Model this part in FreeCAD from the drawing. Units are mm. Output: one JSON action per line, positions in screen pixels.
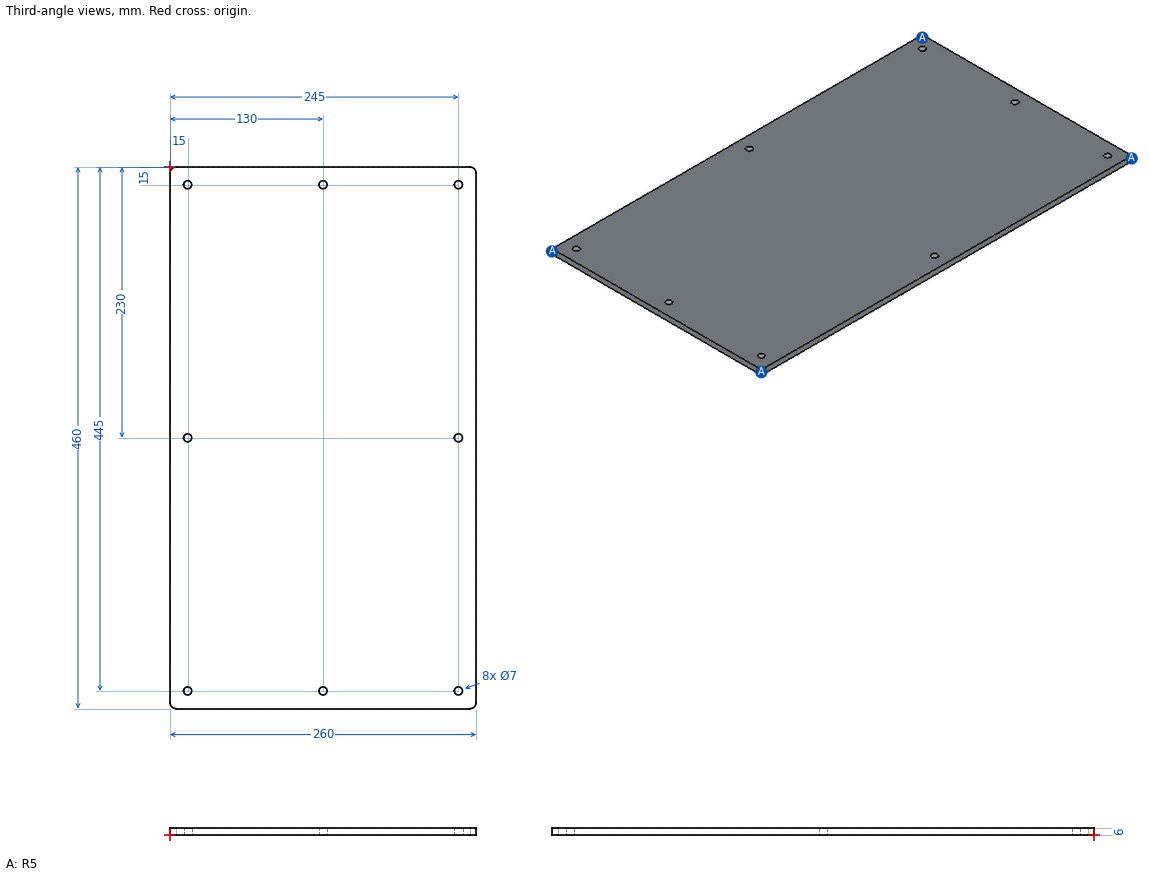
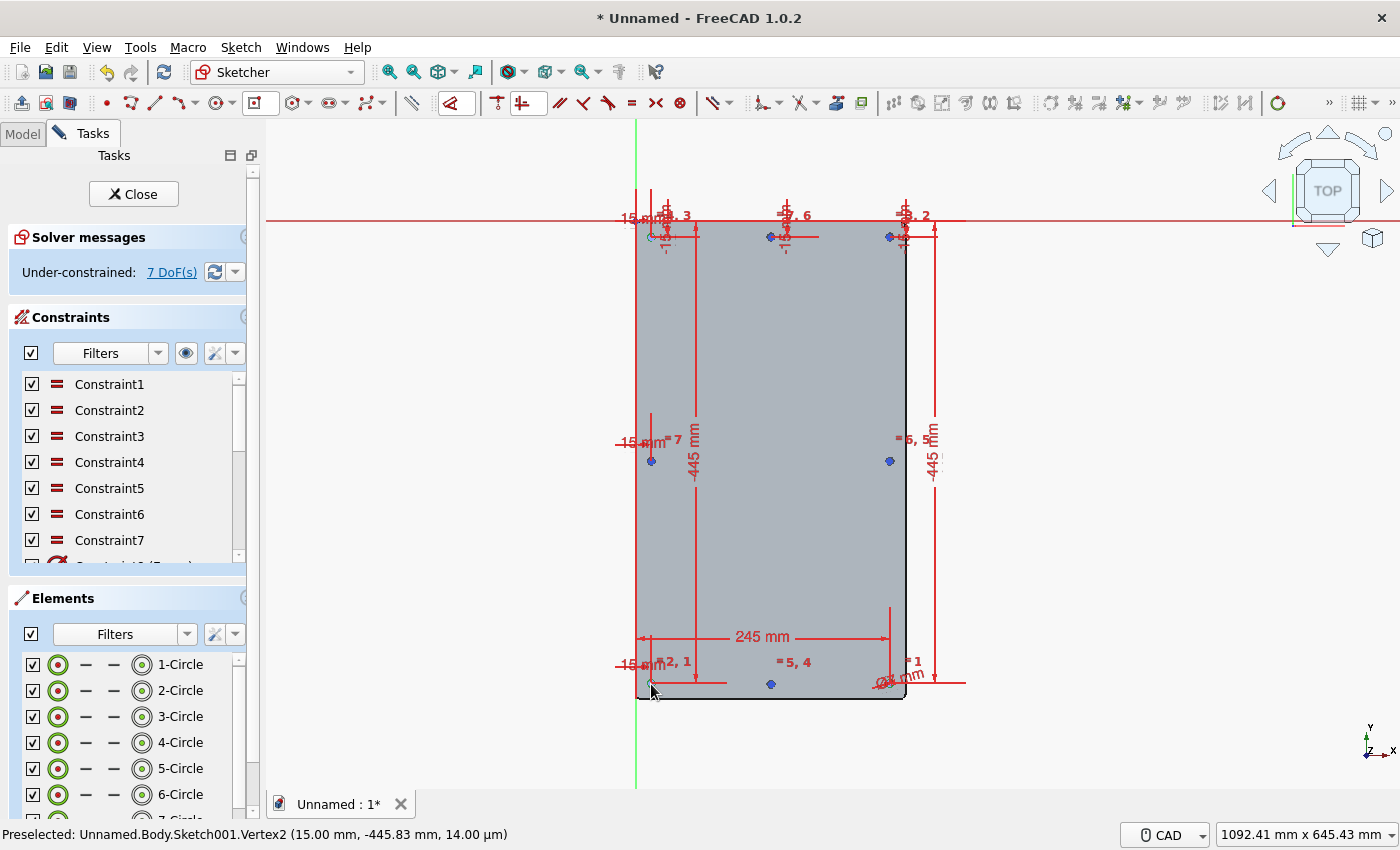
{"action": "left_click", "coordinate": [890, 237]}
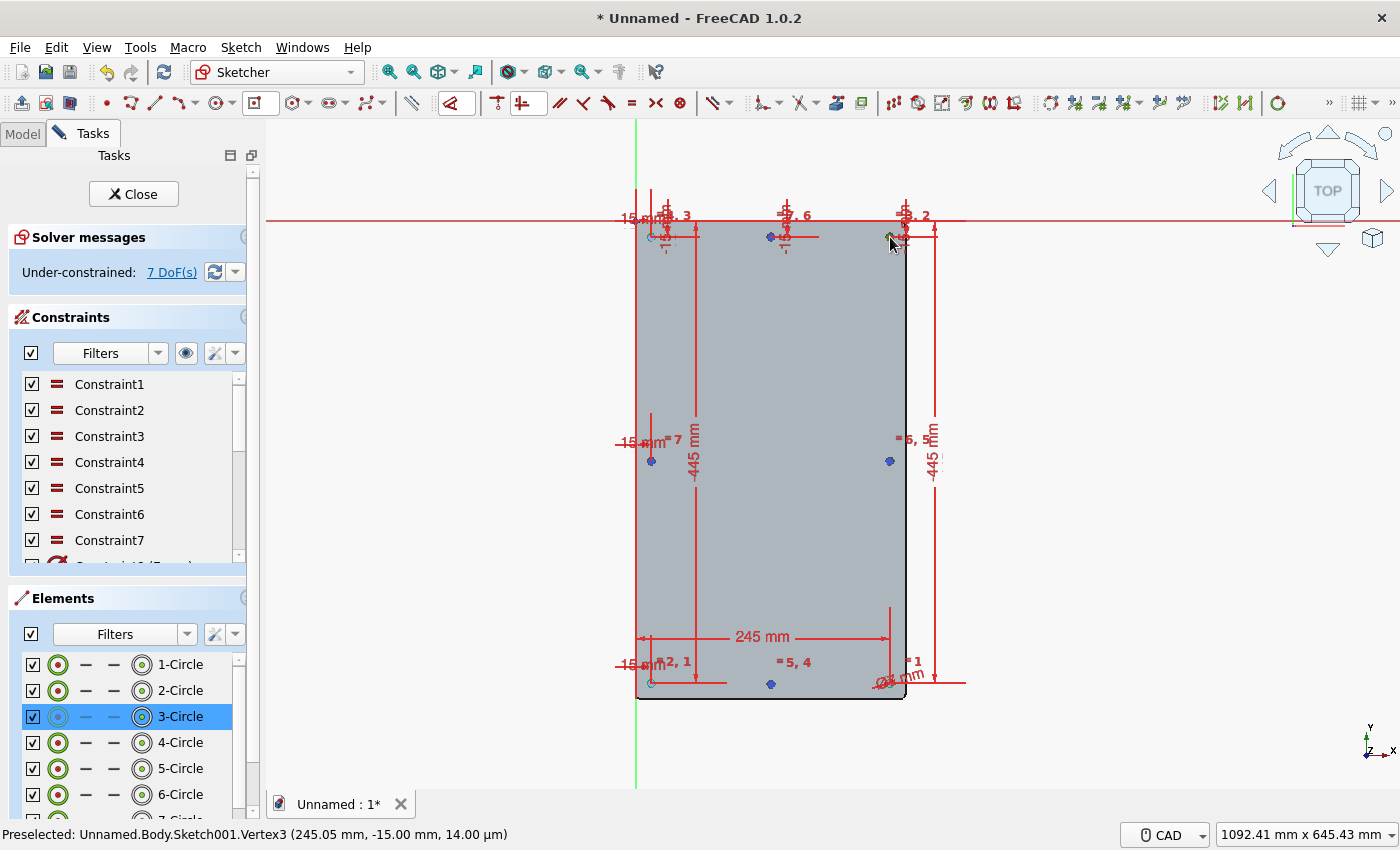
{"action": "key", "text": "l"}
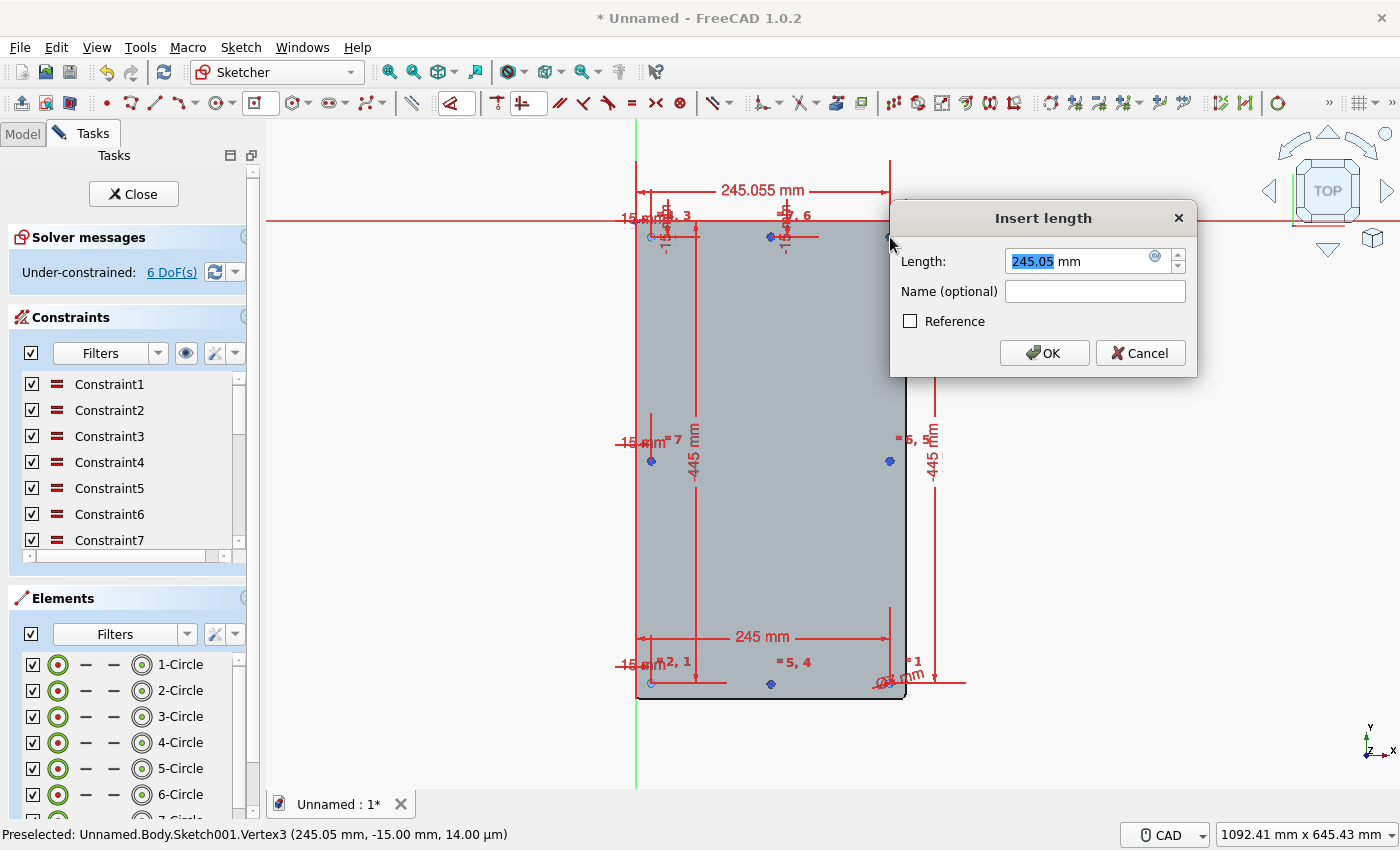
{"action": "type", "text": "245"}
{"action": "key", "text": "Return"}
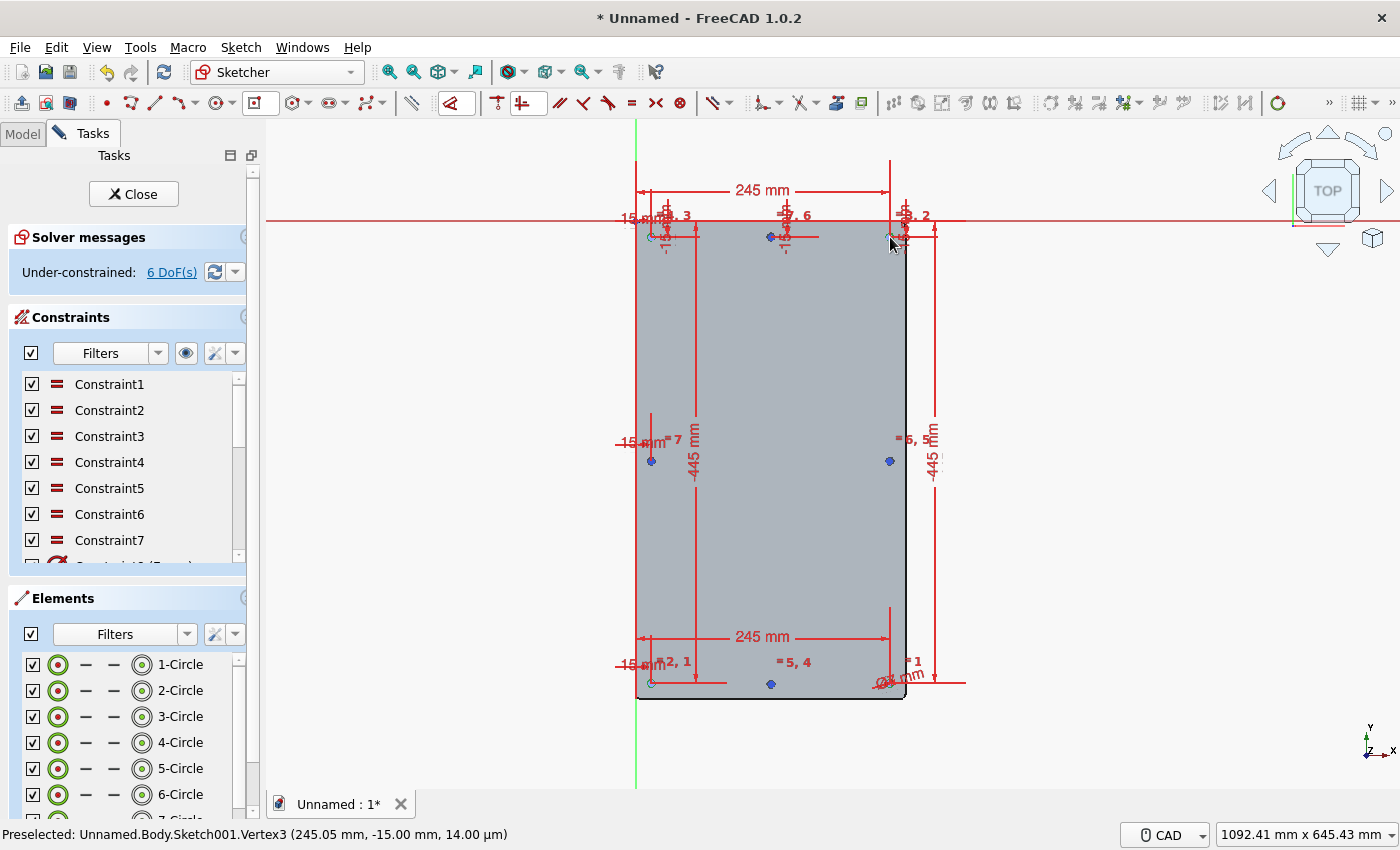
{"action": "left_click", "coordinate": [771, 684]}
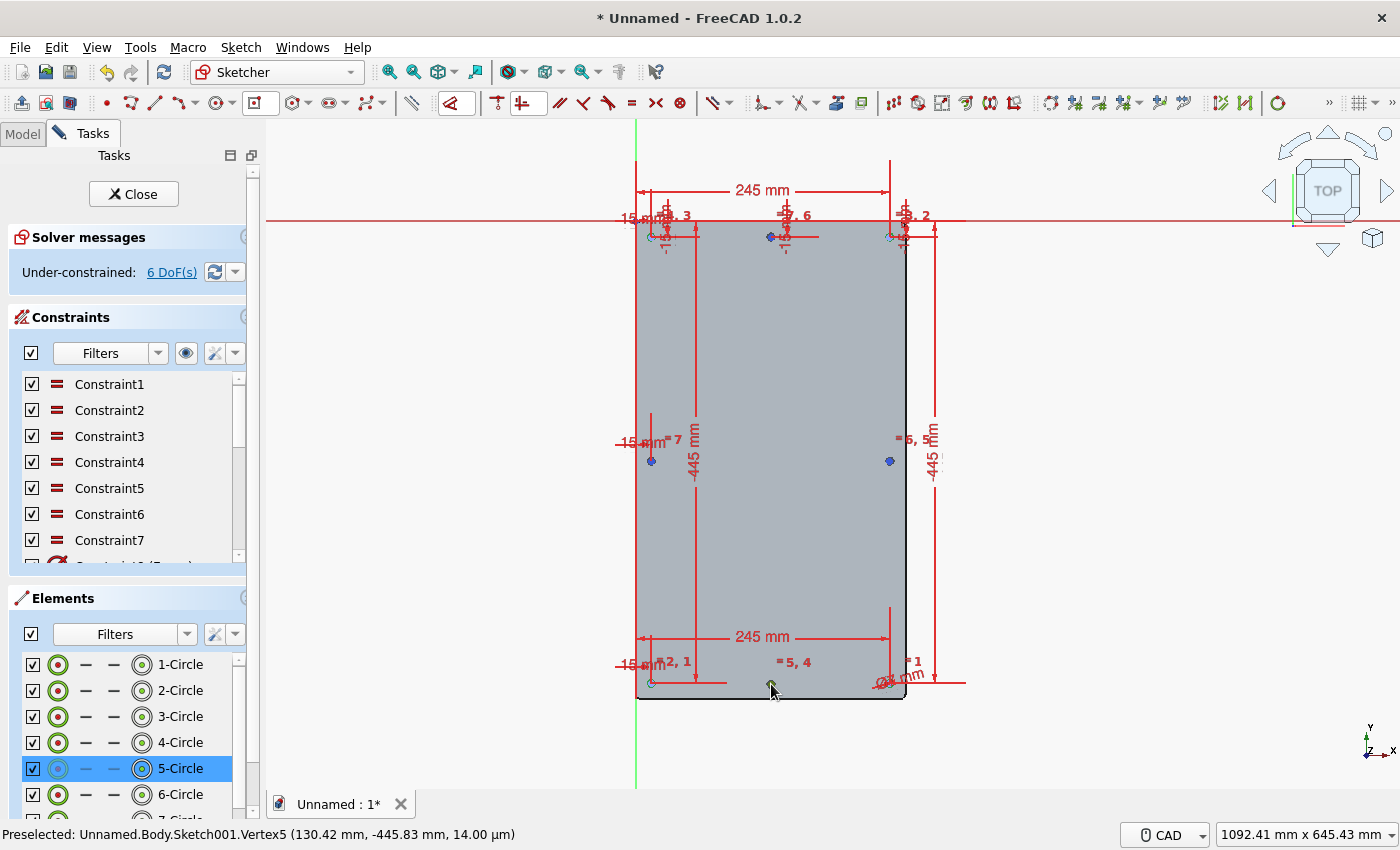
{"action": "key", "text": "l"}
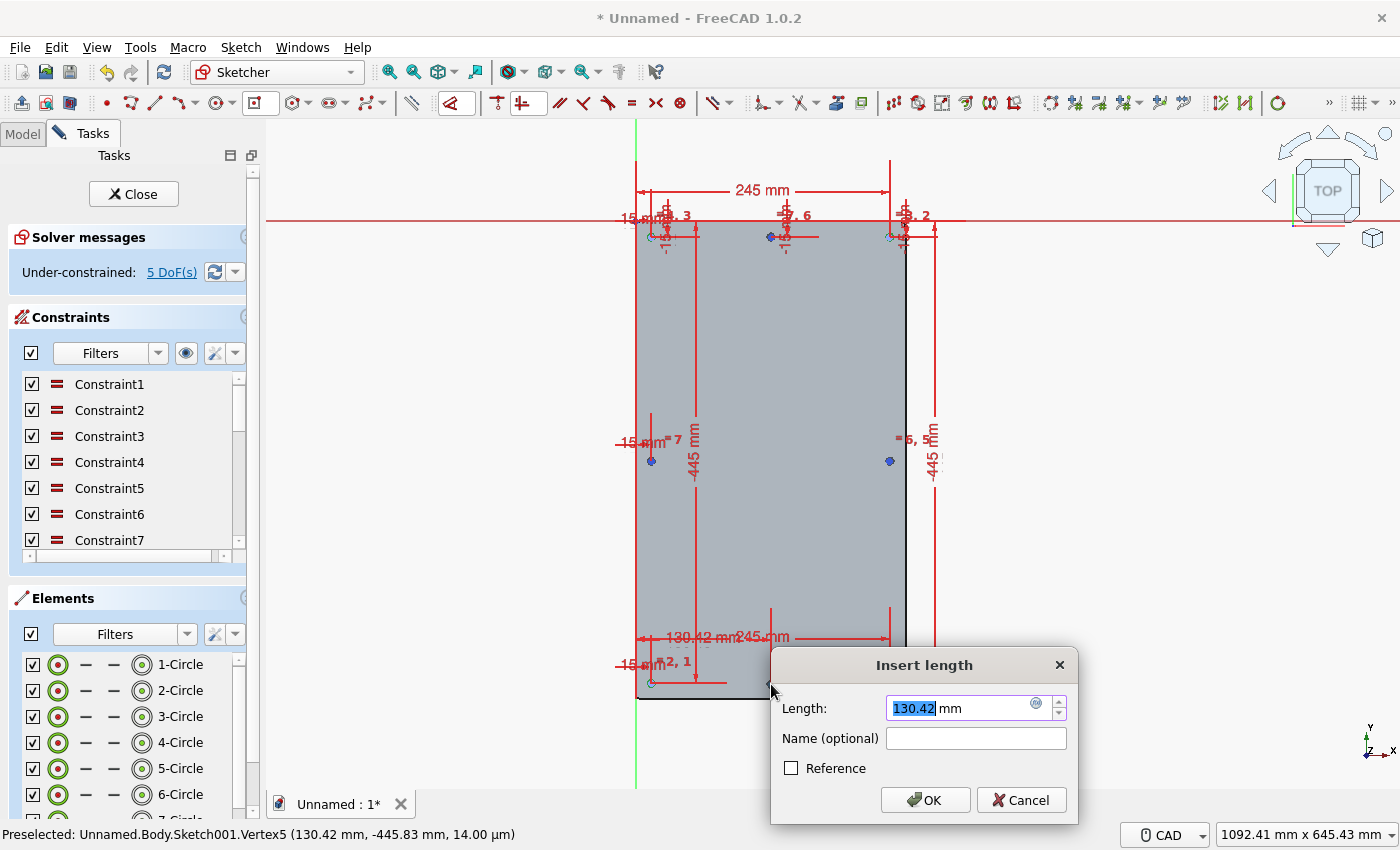
{"action": "type", "text": "130"}
{"action": "key", "text": "Return"}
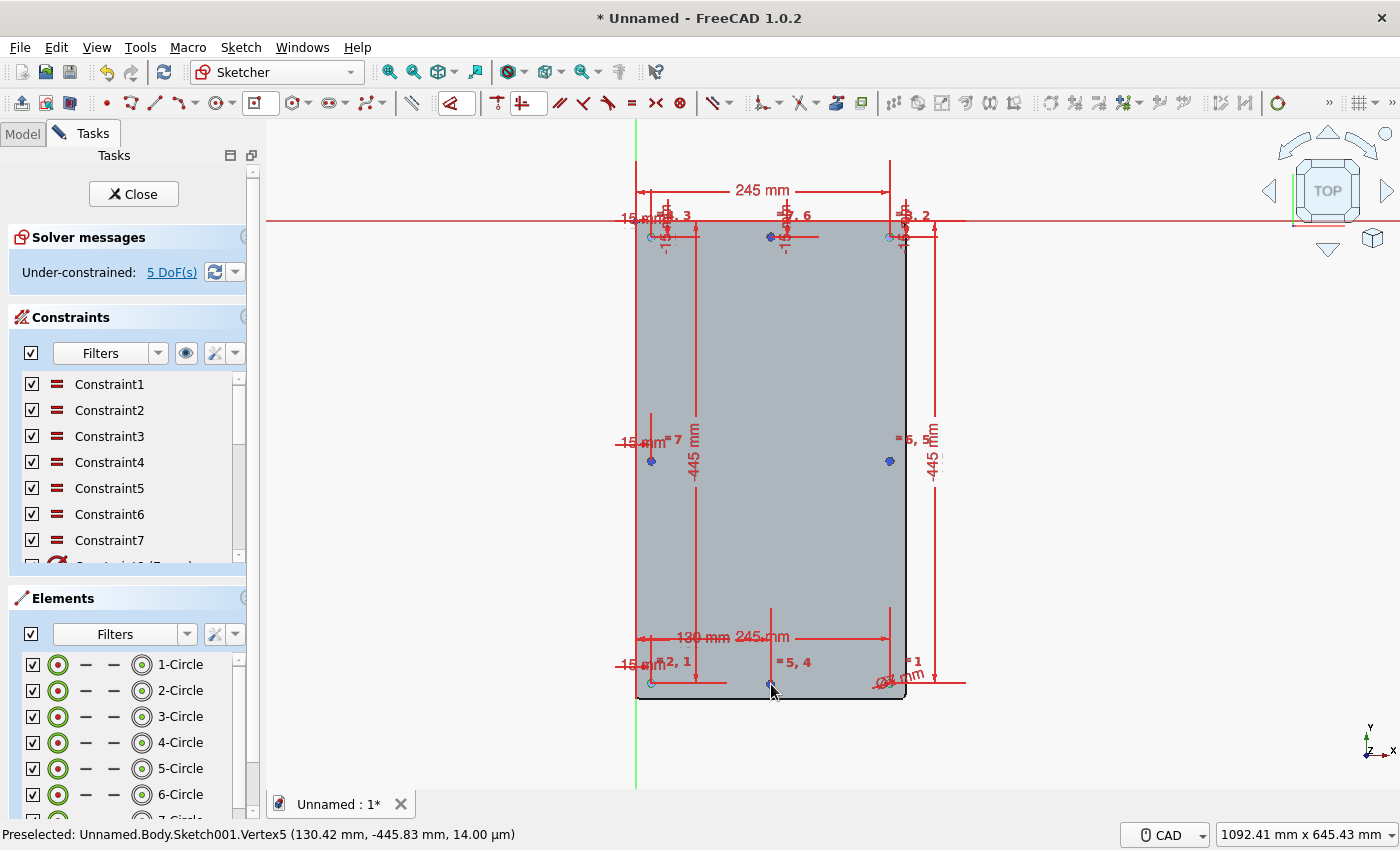
{"action": "left_click", "coordinate": [771, 684]}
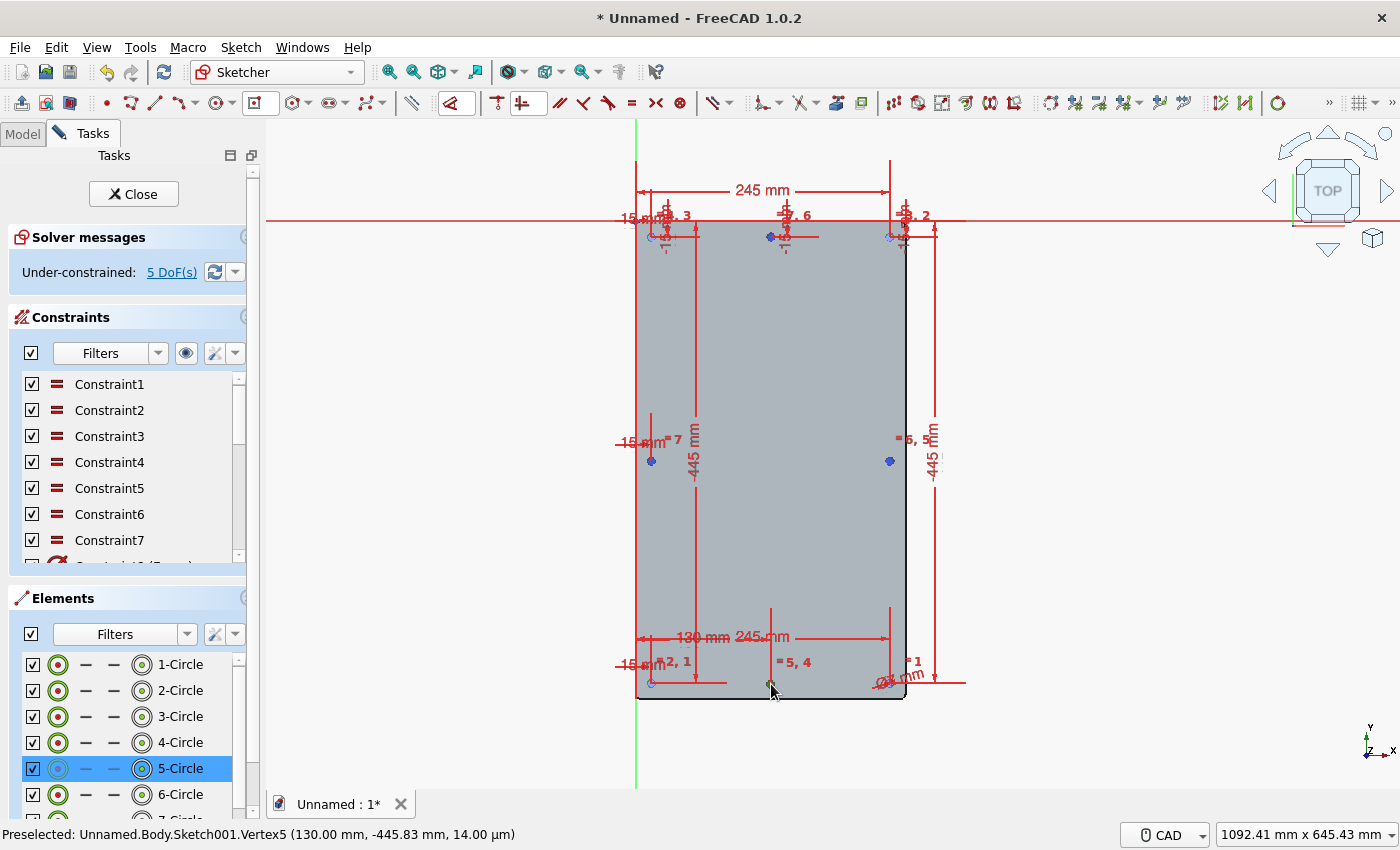
{"action": "left_click", "coordinate": [470, 104]}